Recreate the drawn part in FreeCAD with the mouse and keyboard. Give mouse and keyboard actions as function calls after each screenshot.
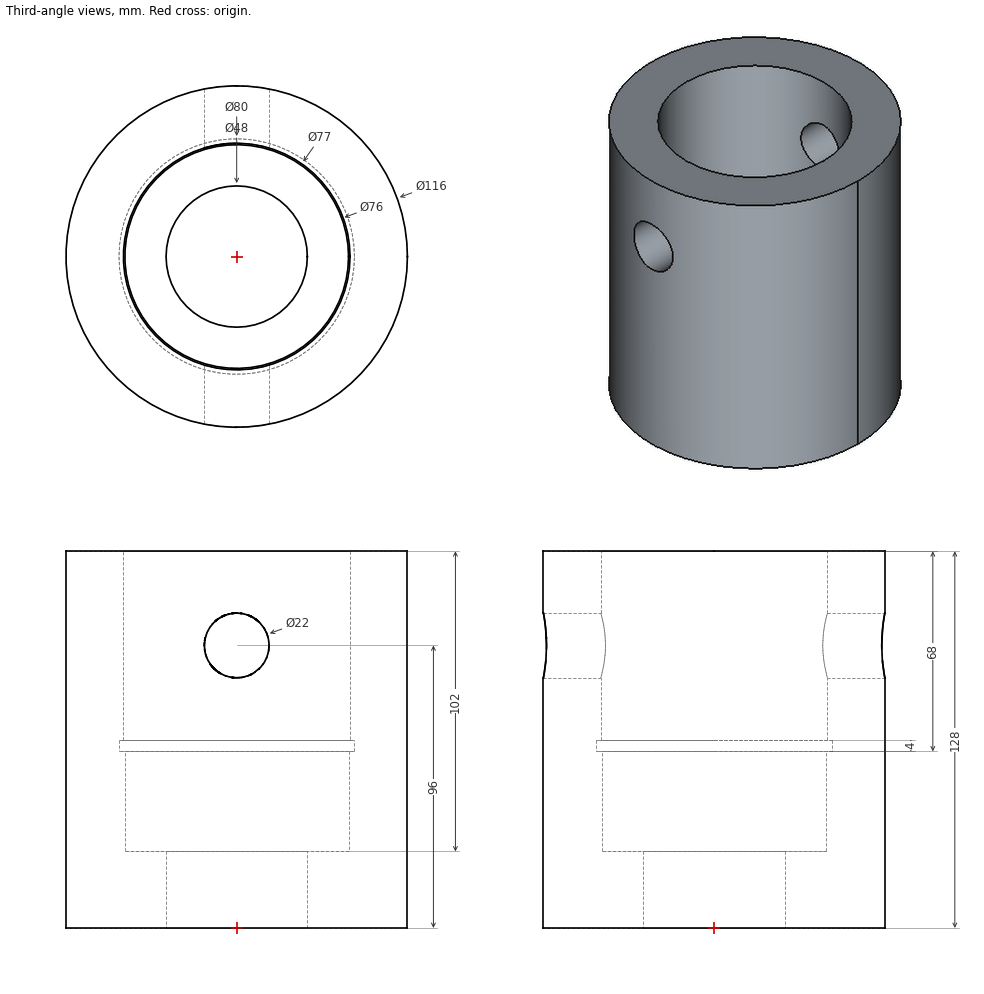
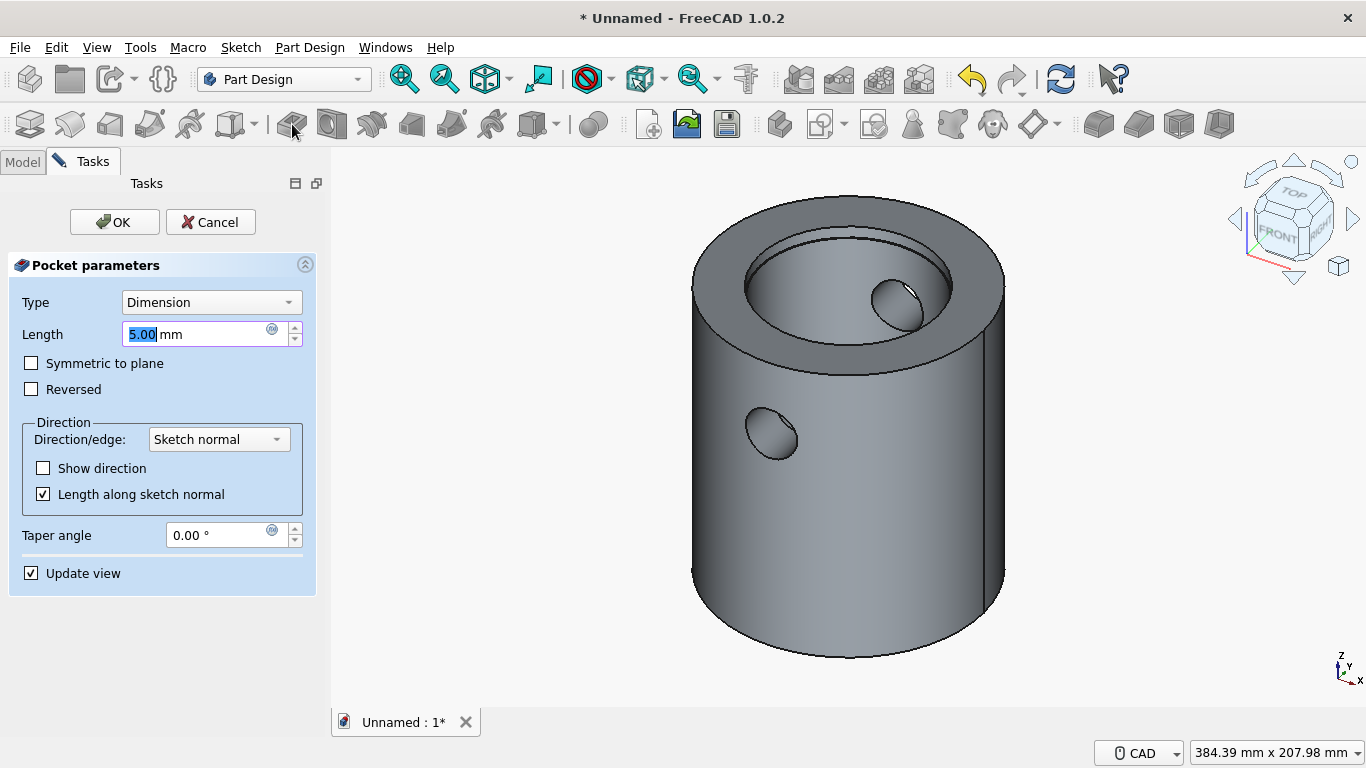
text(68)
key(Tab)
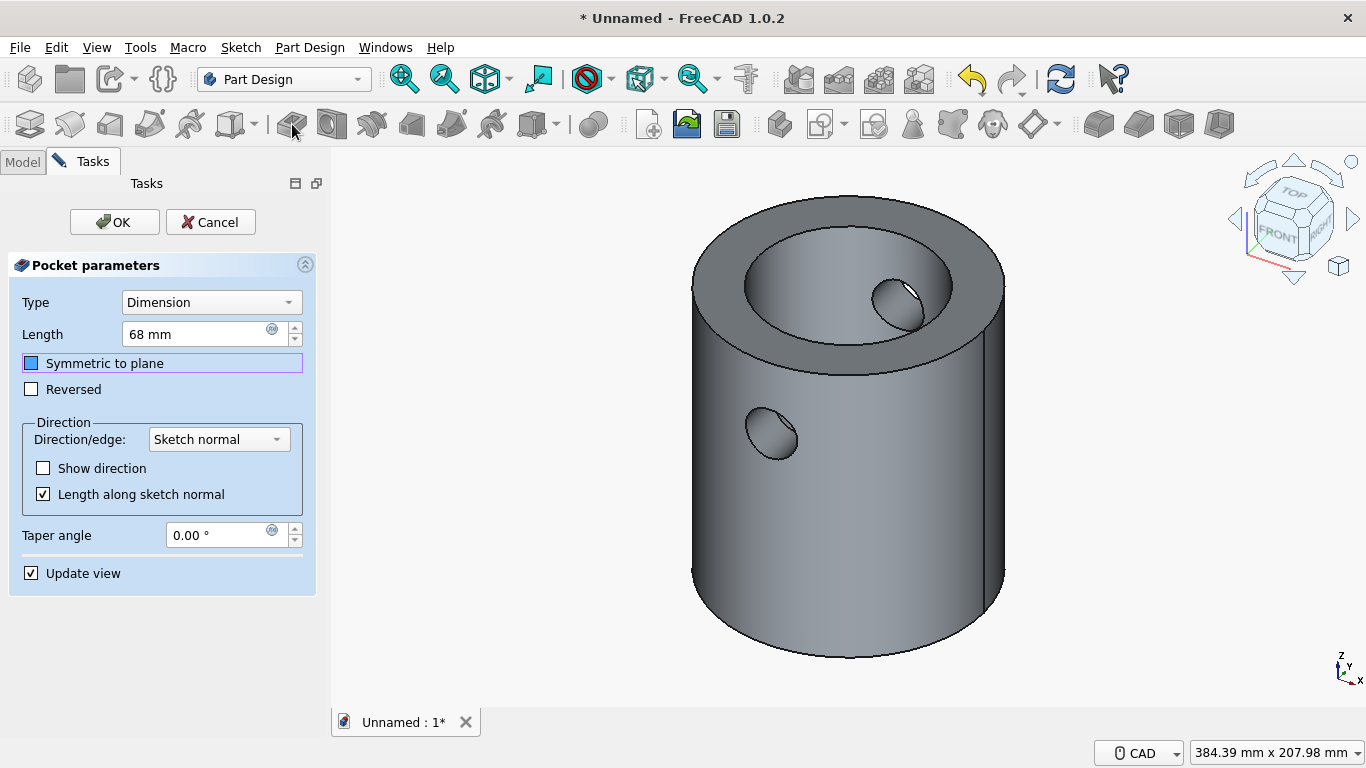
click(115, 222)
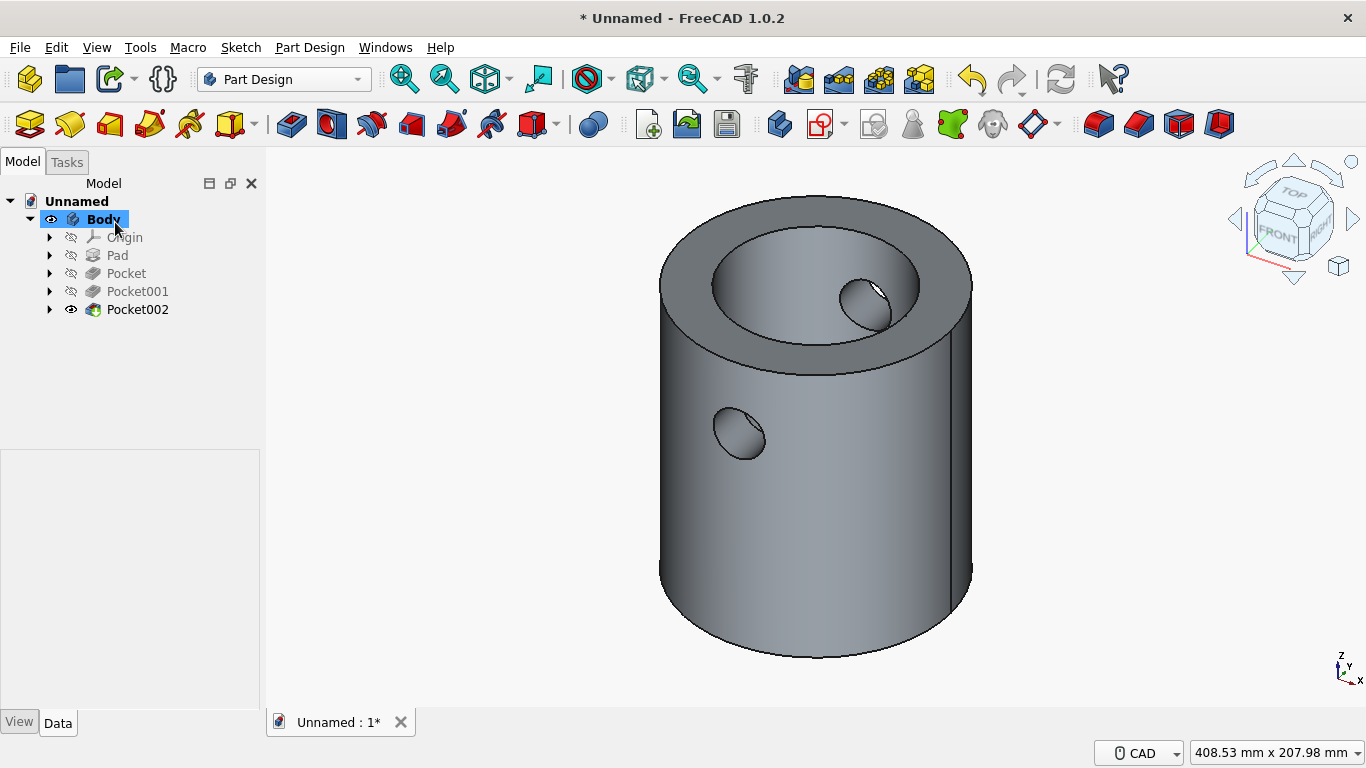
scroll(714, 444, up, 15)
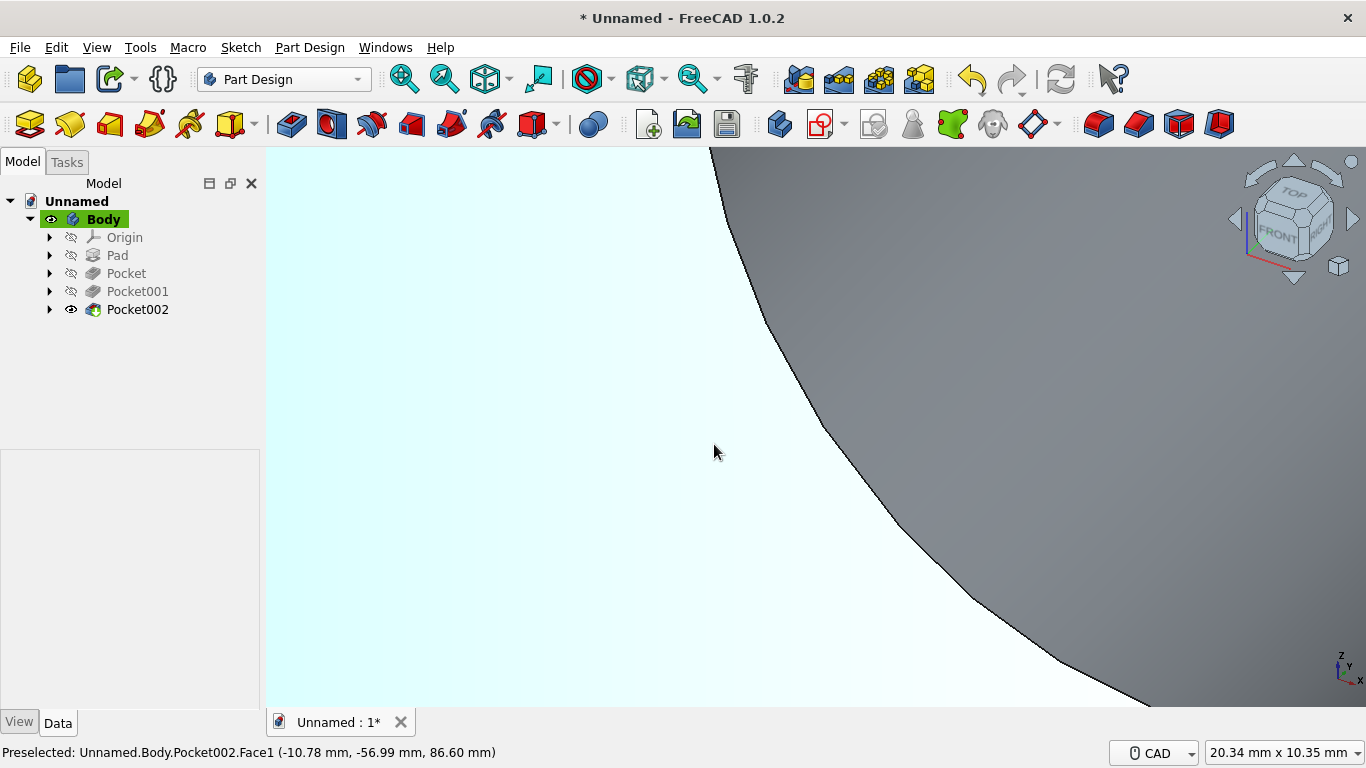
click(406, 80)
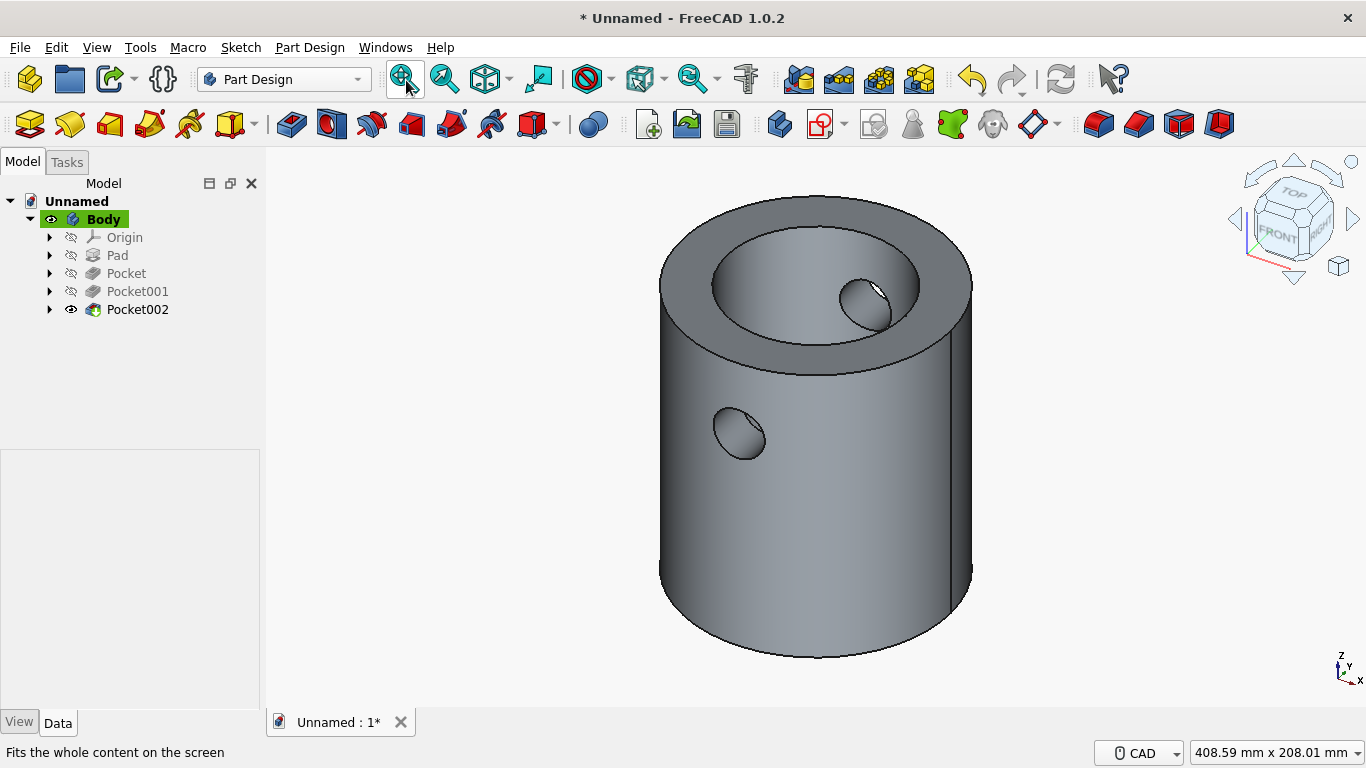
key(0)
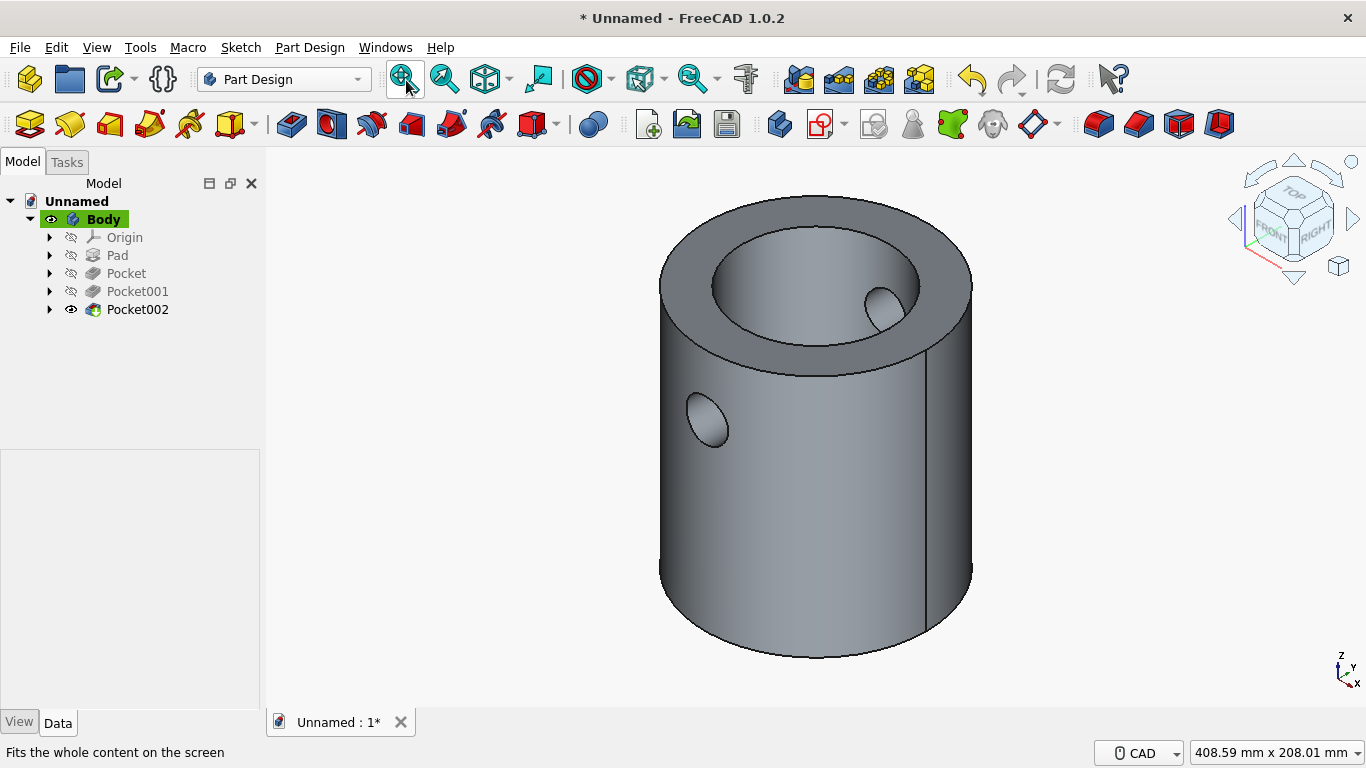
scroll(713, 429, up, 15)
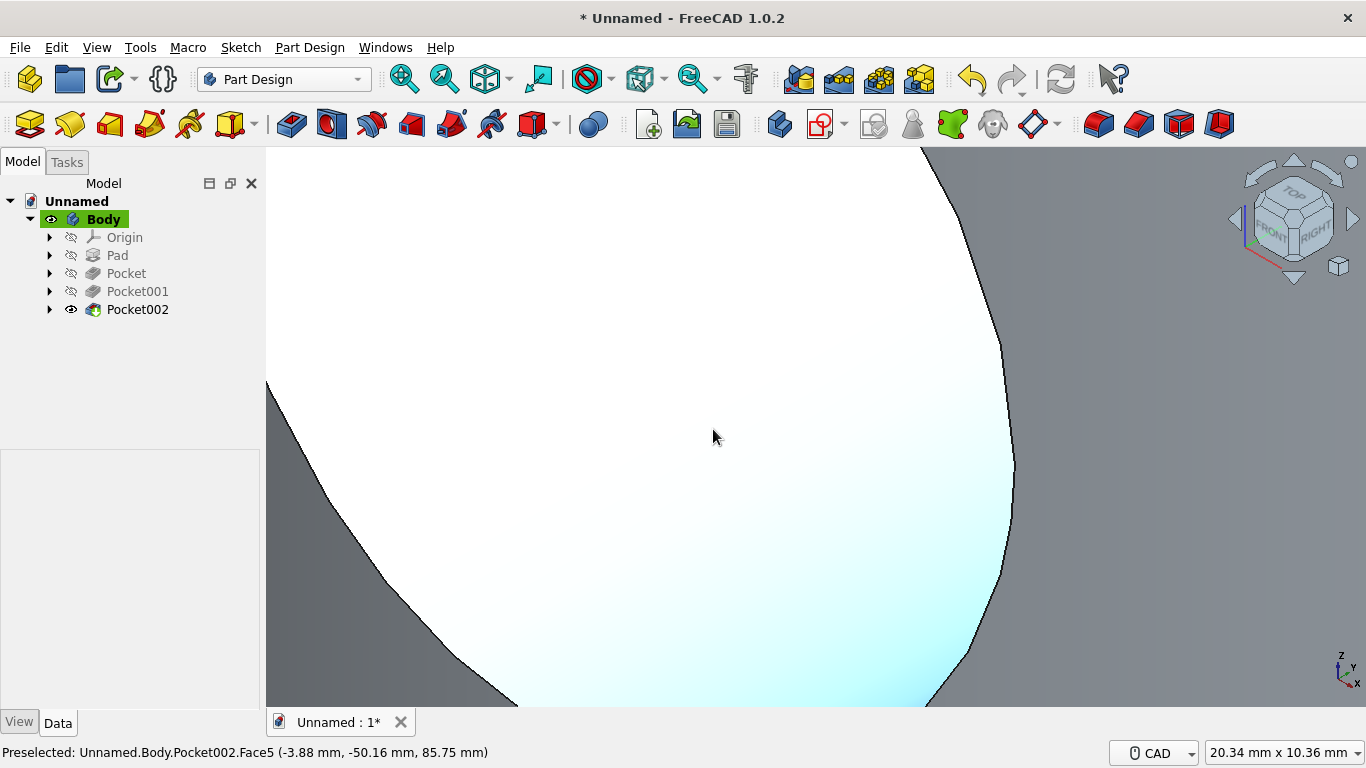
click(406, 80)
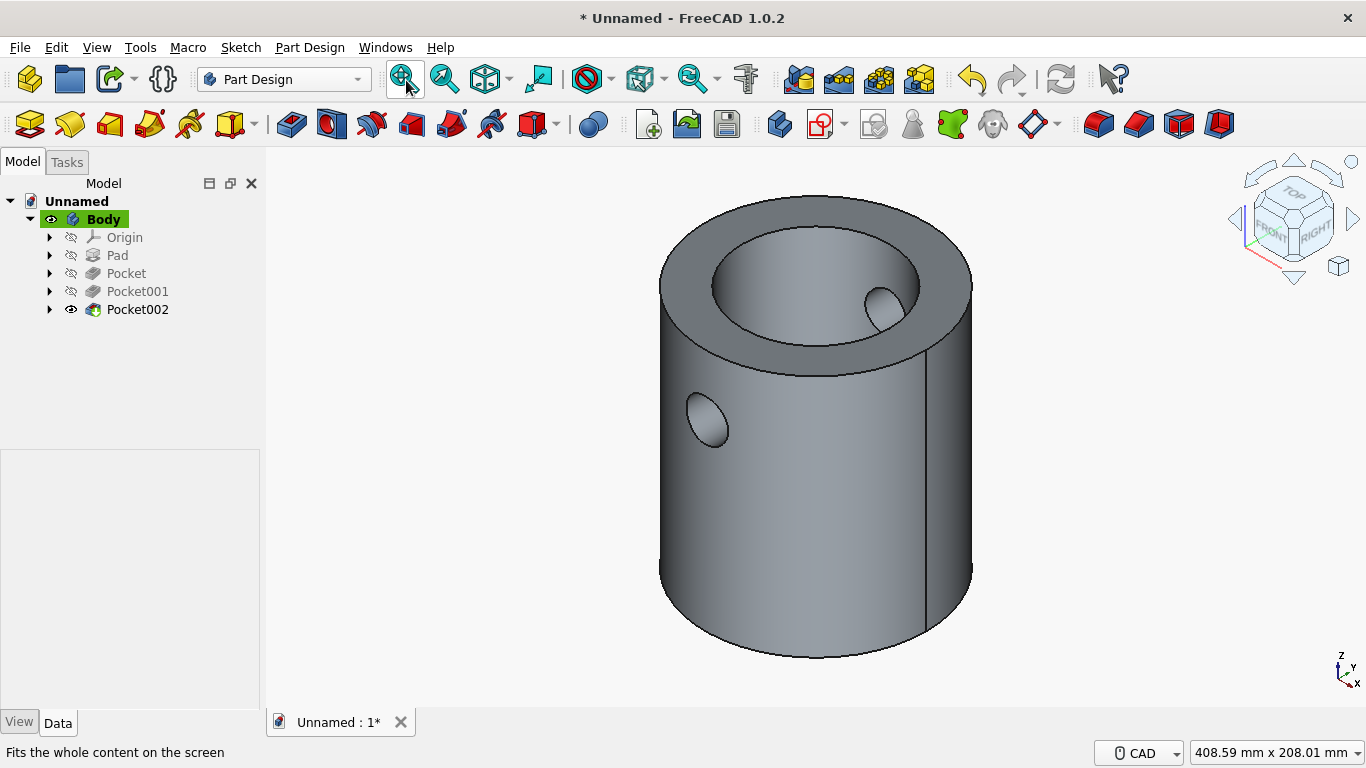
key(2)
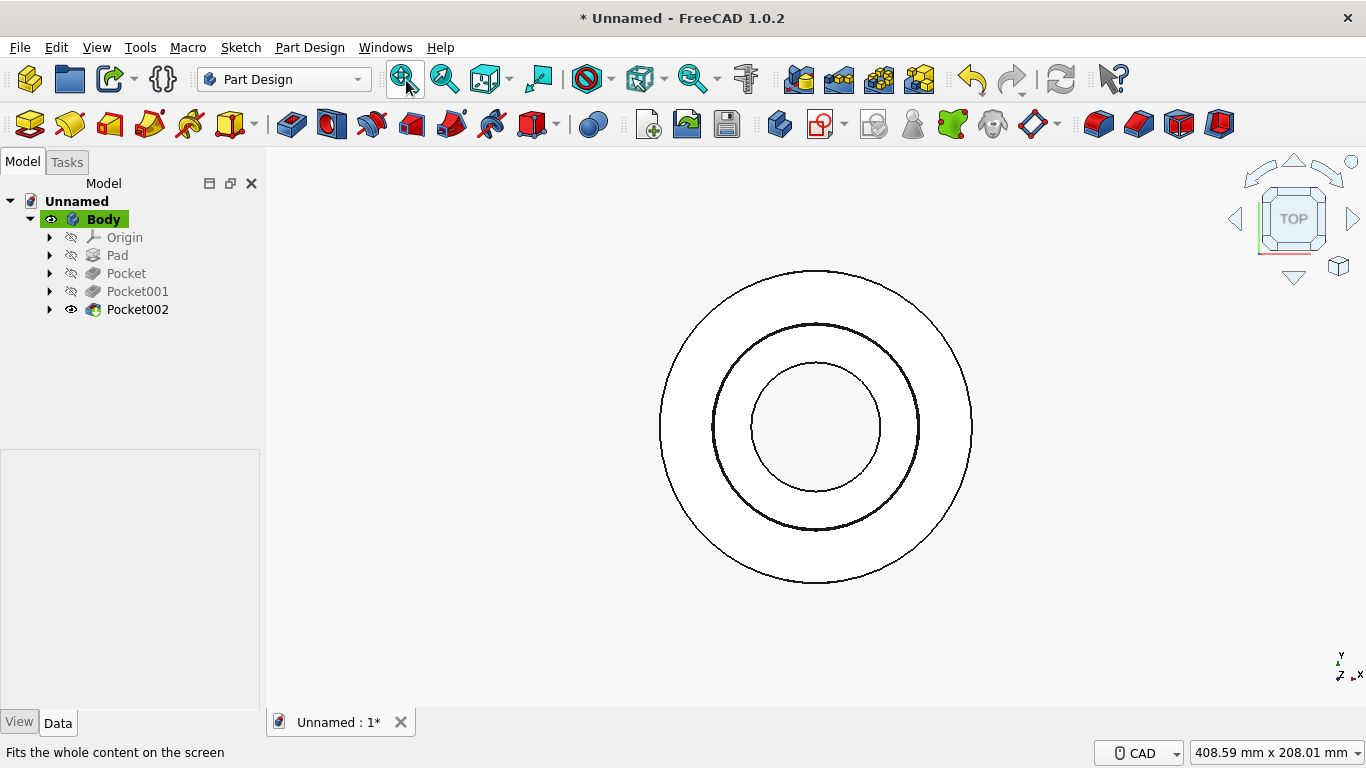
scroll(736, 491, up, 15)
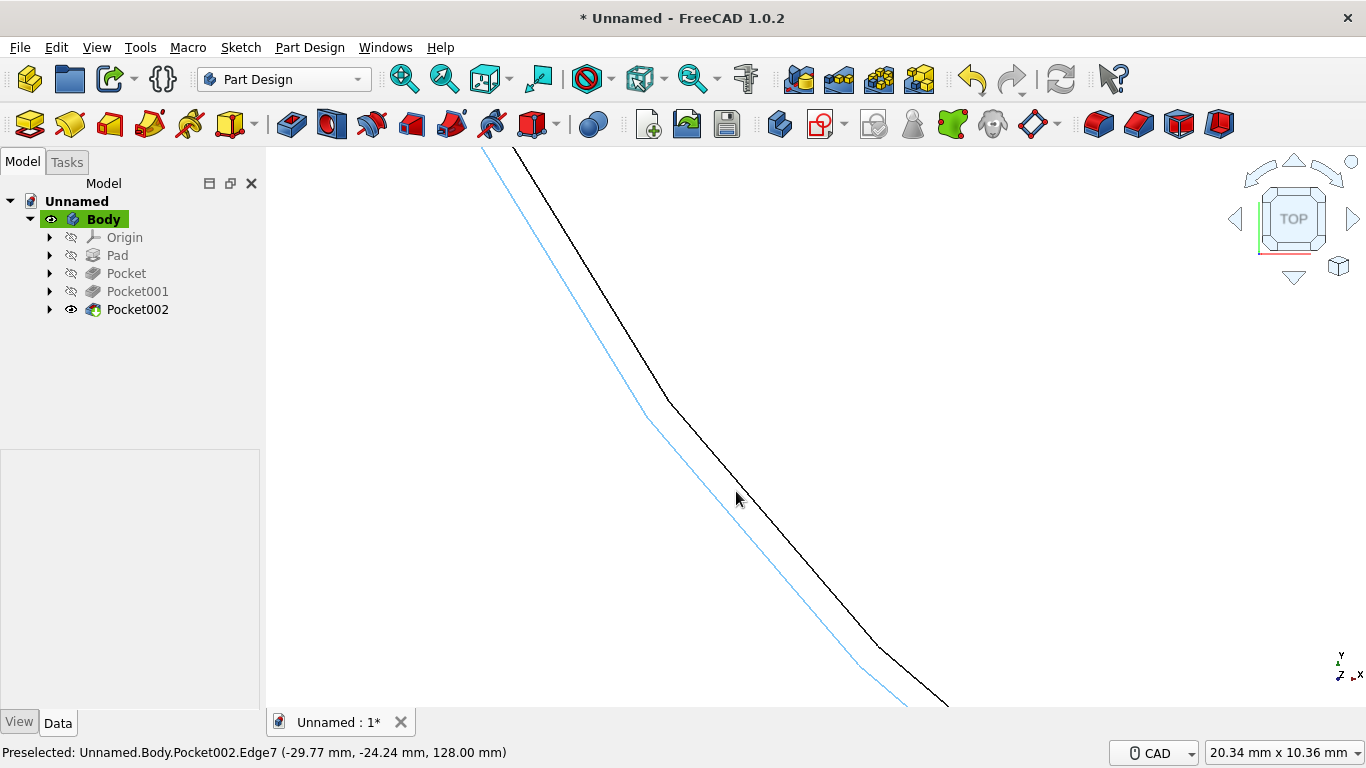
click(406, 80)